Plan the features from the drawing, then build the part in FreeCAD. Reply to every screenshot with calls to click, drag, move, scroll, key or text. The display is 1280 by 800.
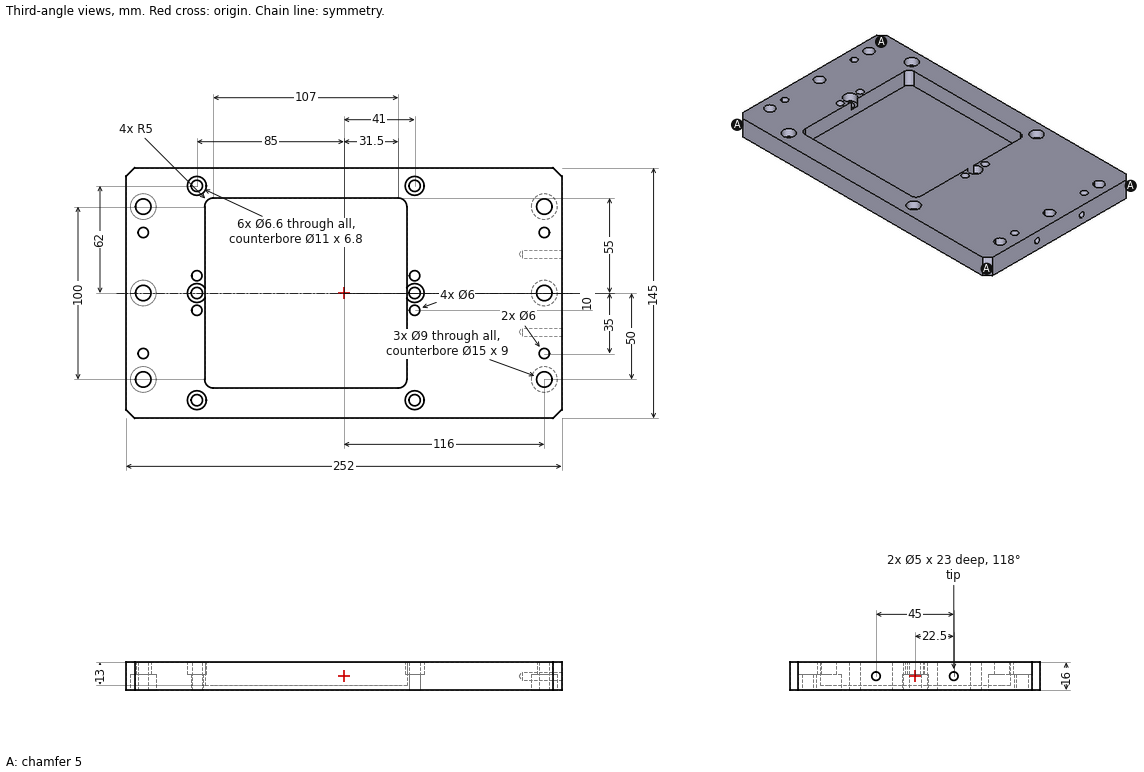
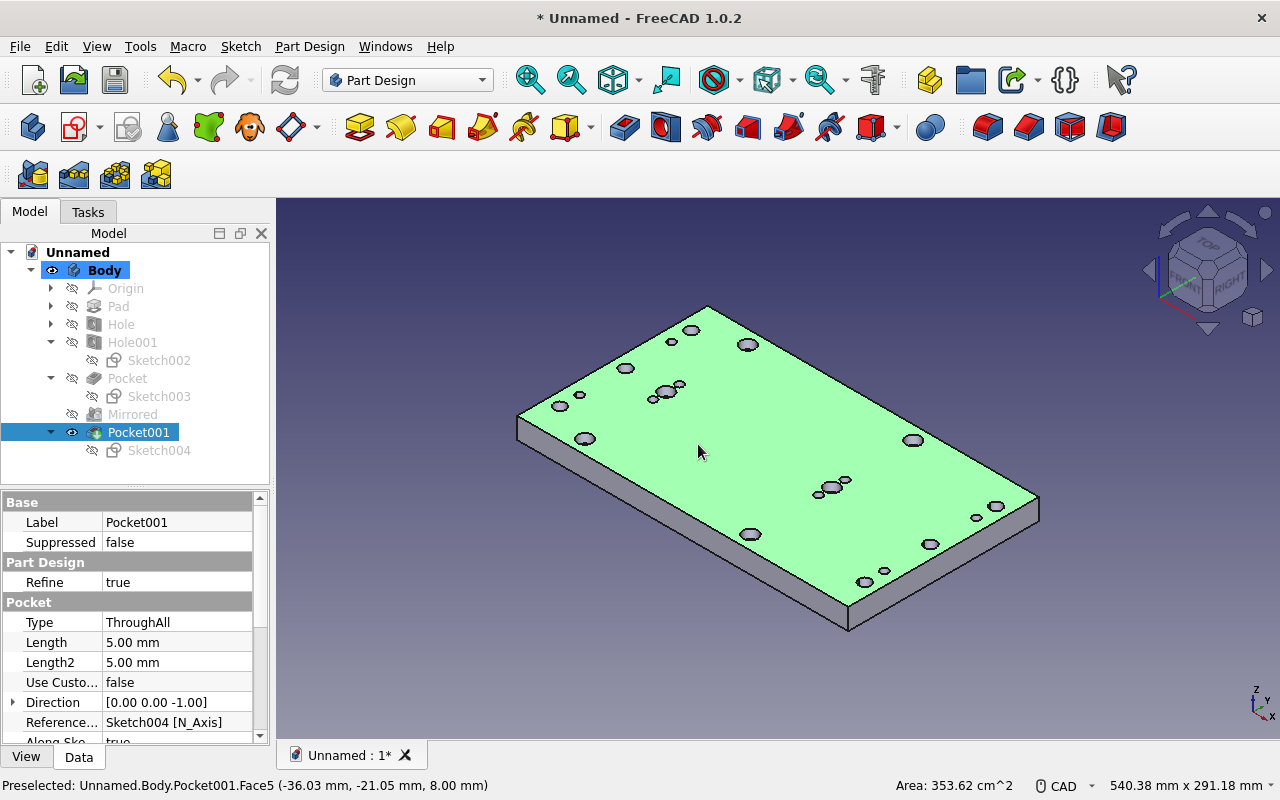
click(74, 128)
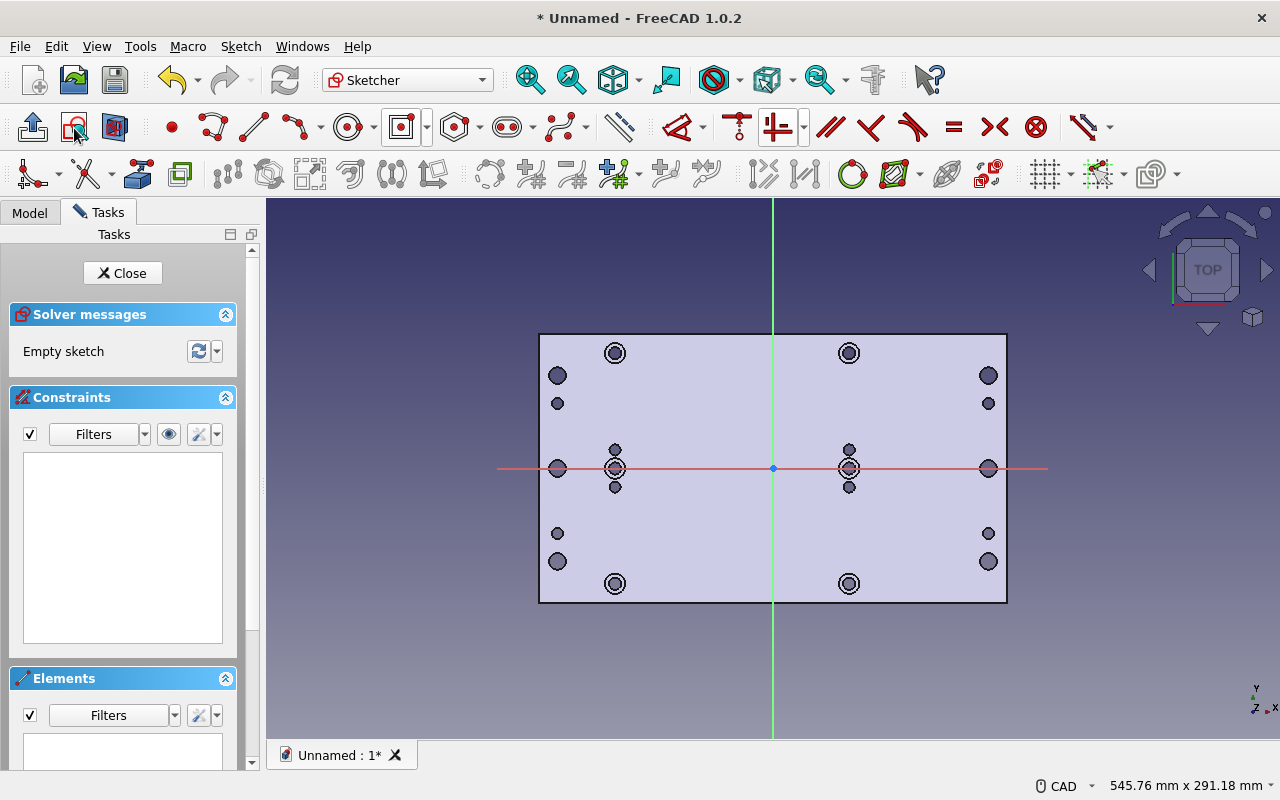
scroll(766, 468, up, 3)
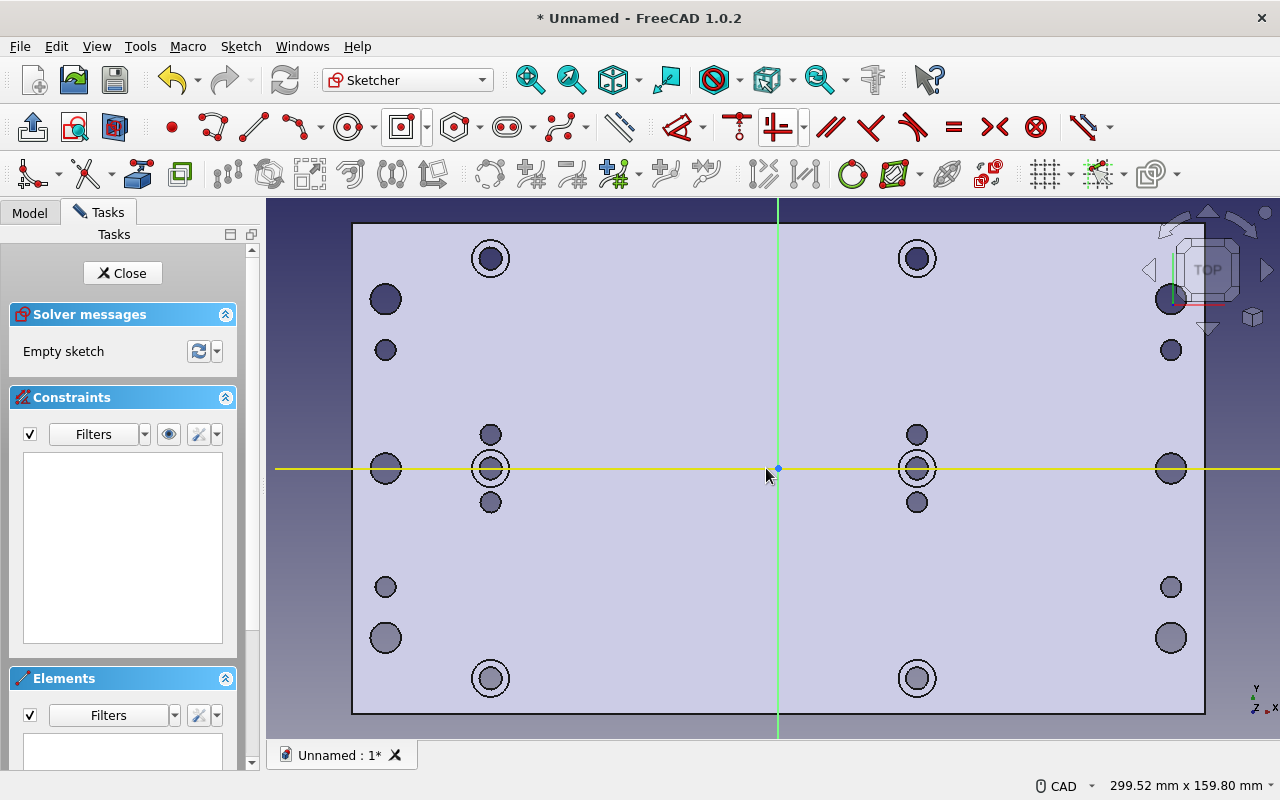
click(254, 128)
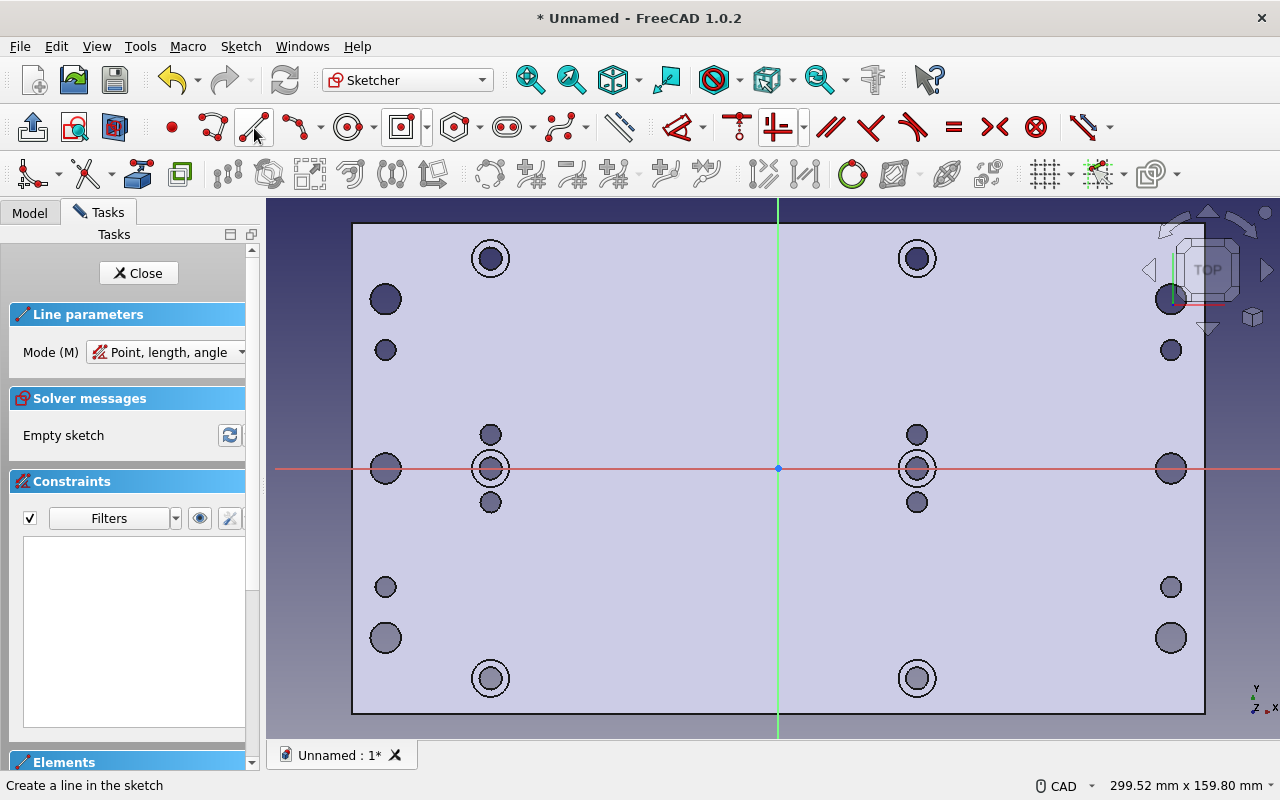
click(885, 282)
click(523, 282)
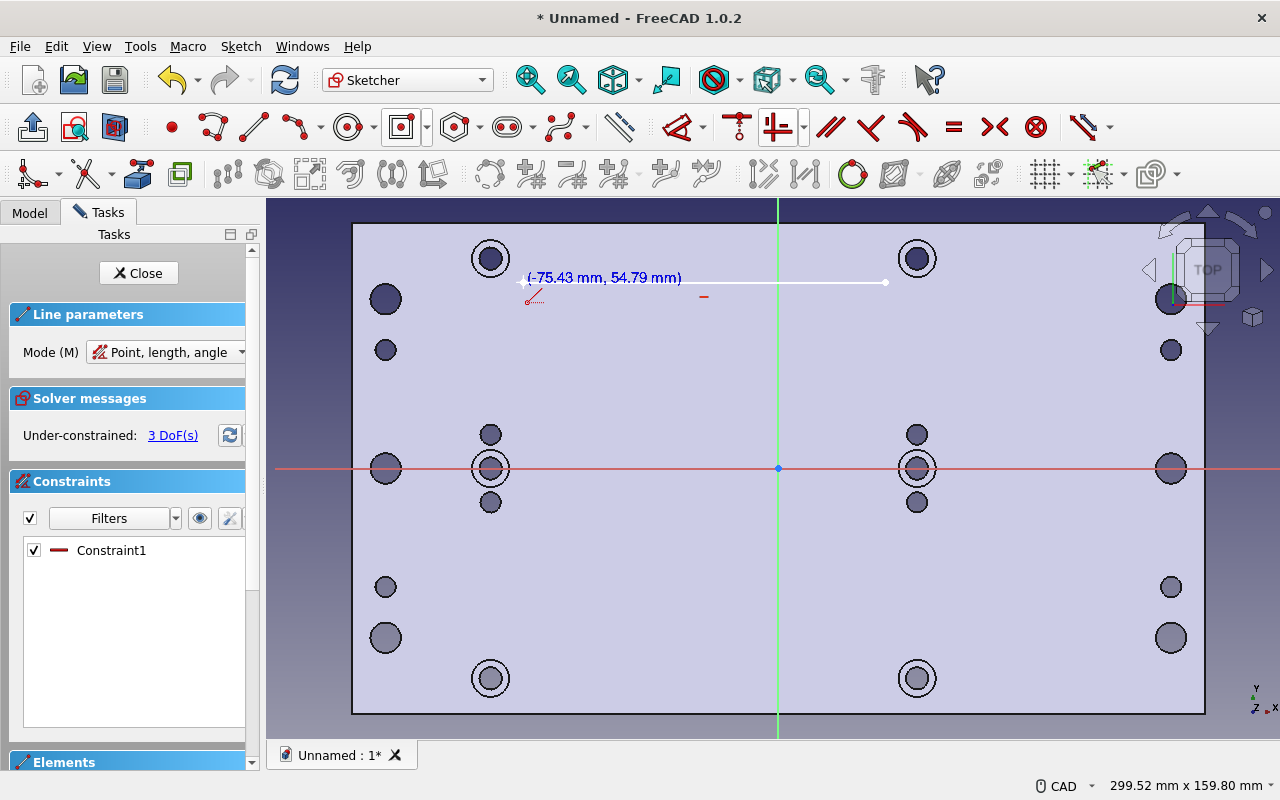
click(506, 299)
click(506, 638)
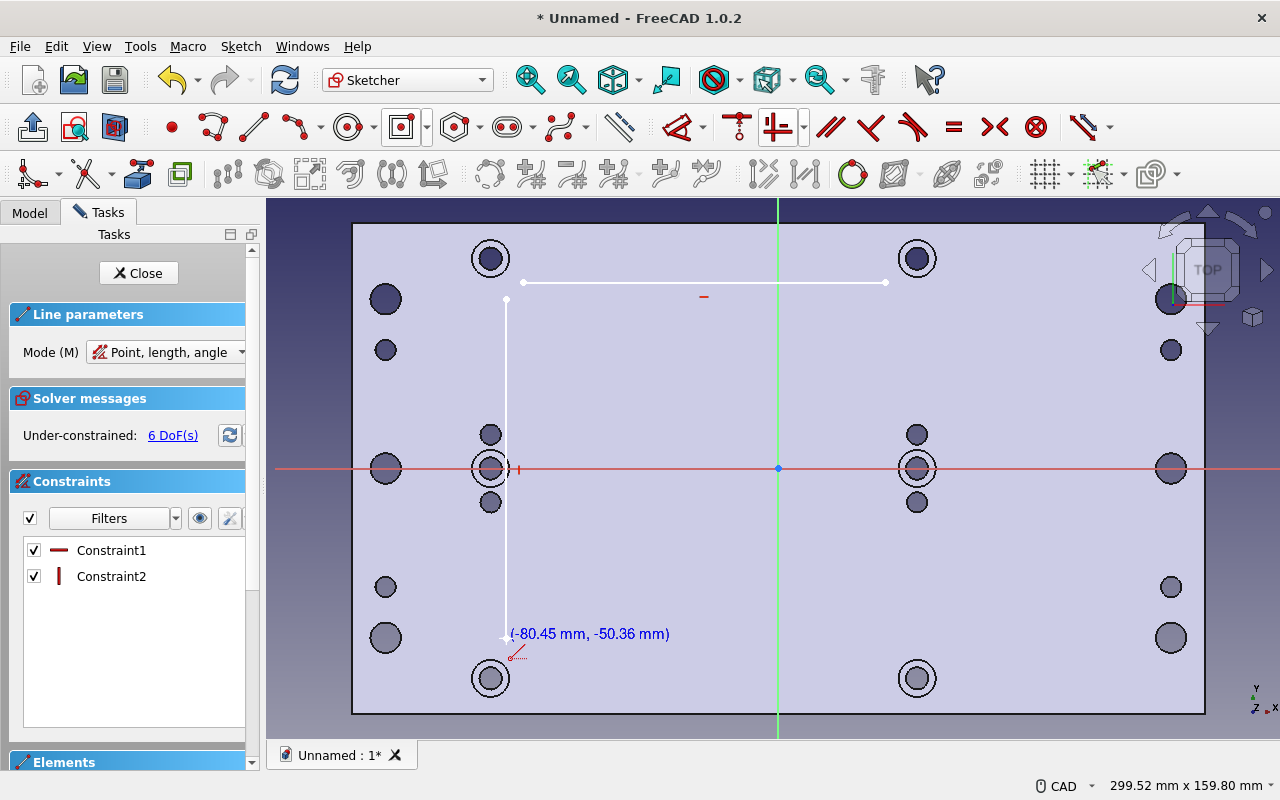
click(523, 655)
click(885, 655)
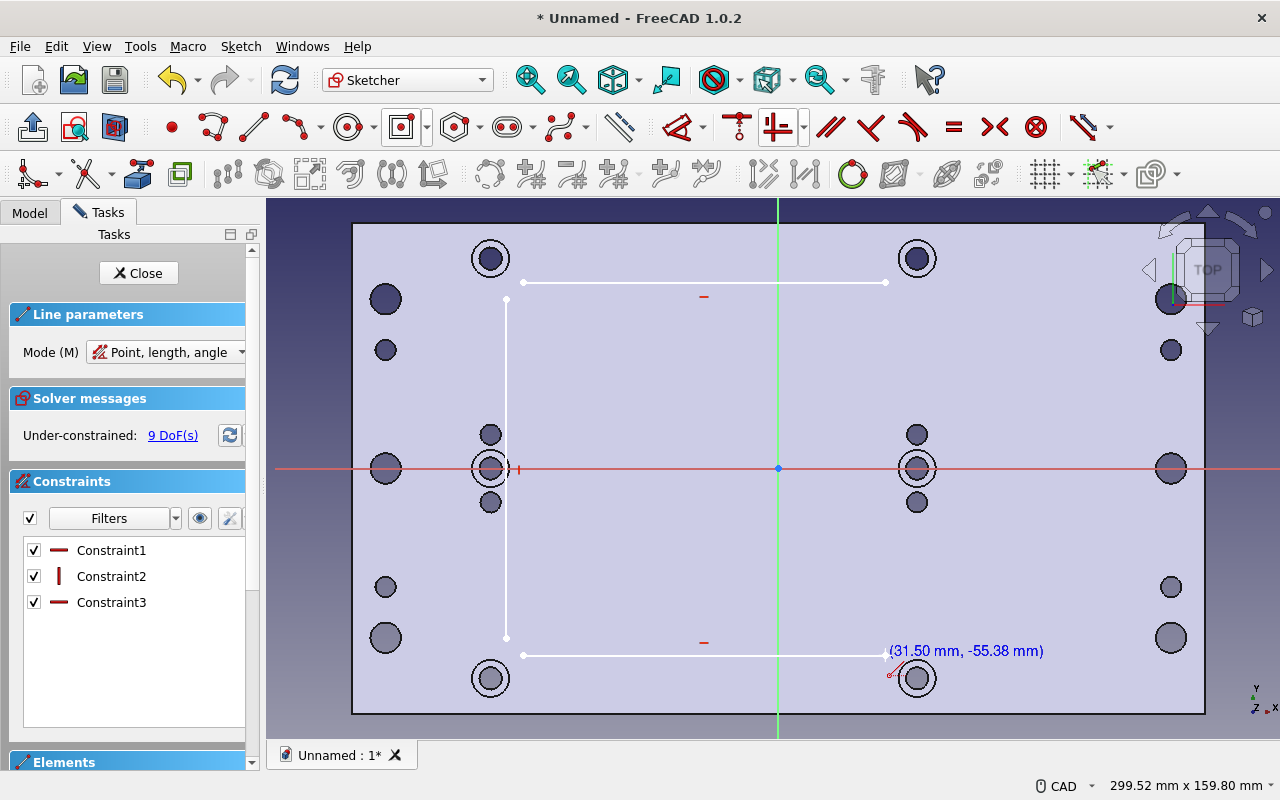
click(902, 638)
click(902, 299)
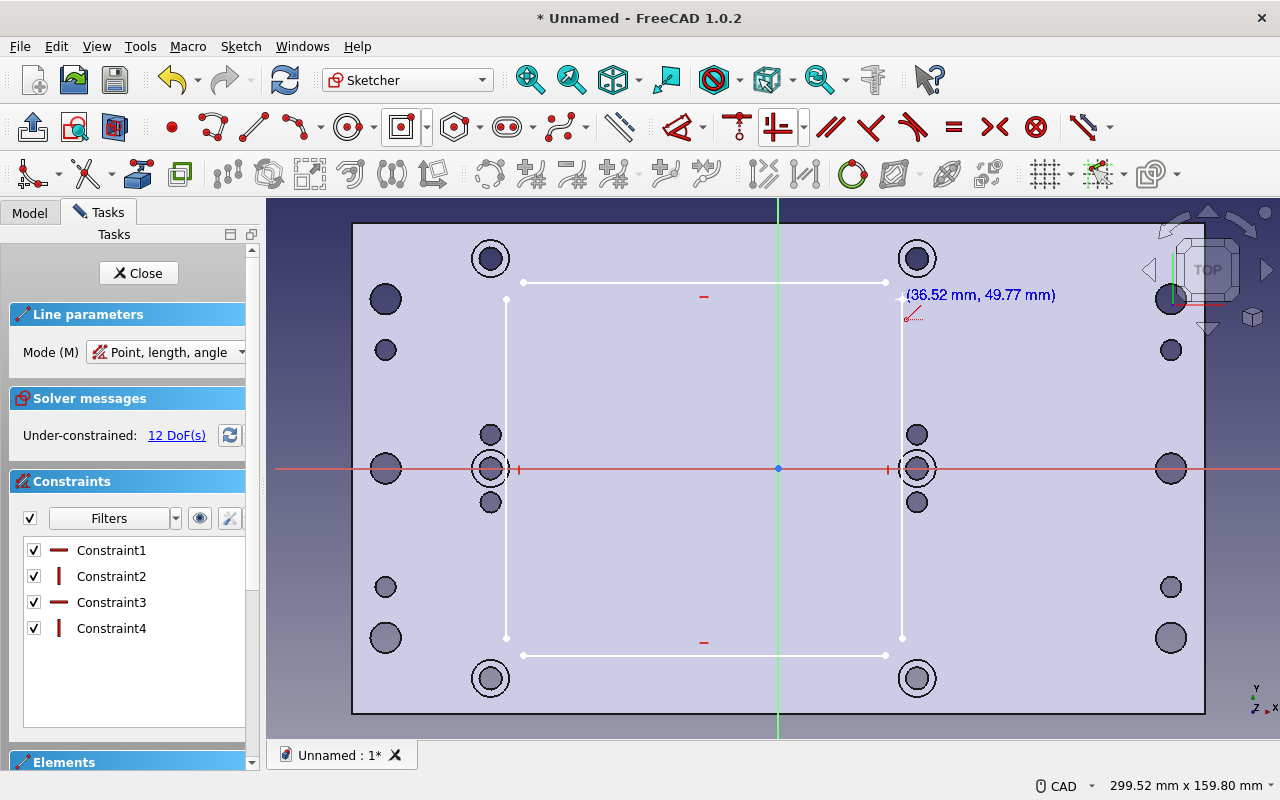
key(g)
key(3)
key(a)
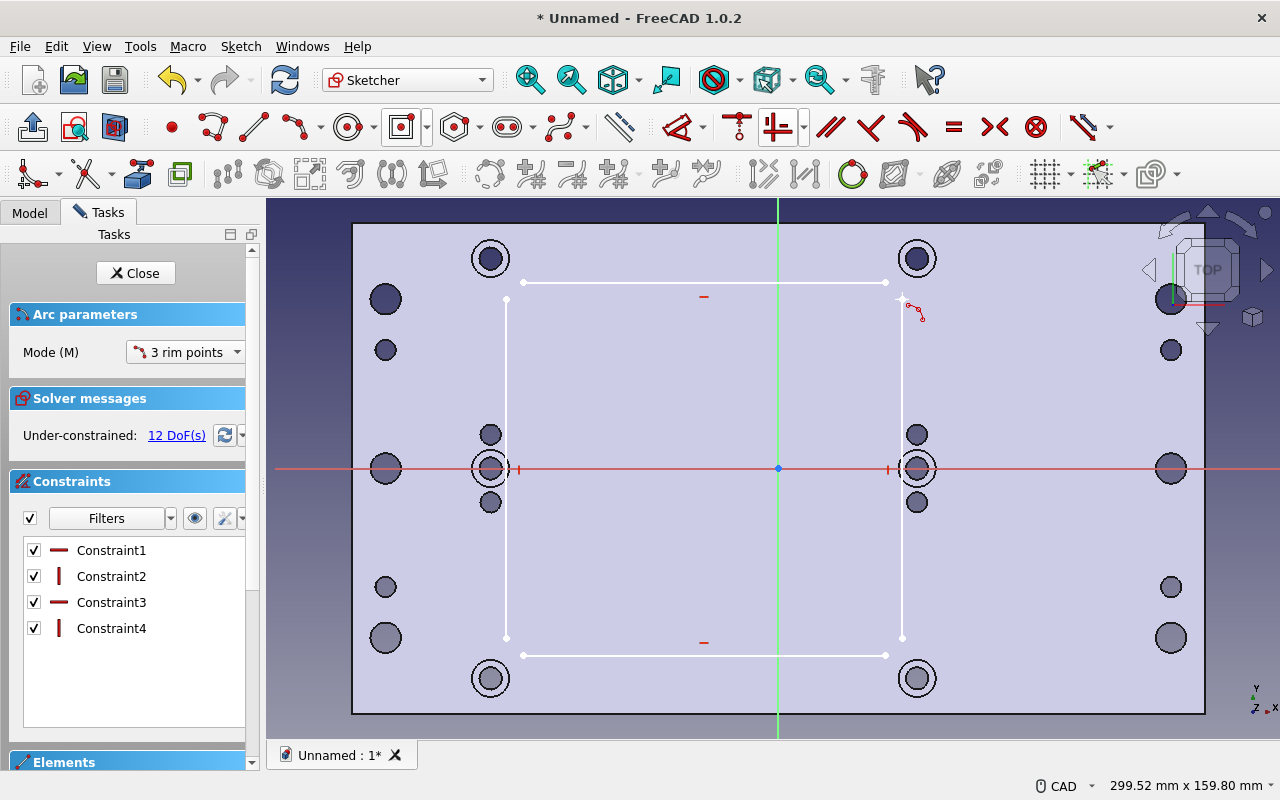
click(523, 283)
click(506, 300)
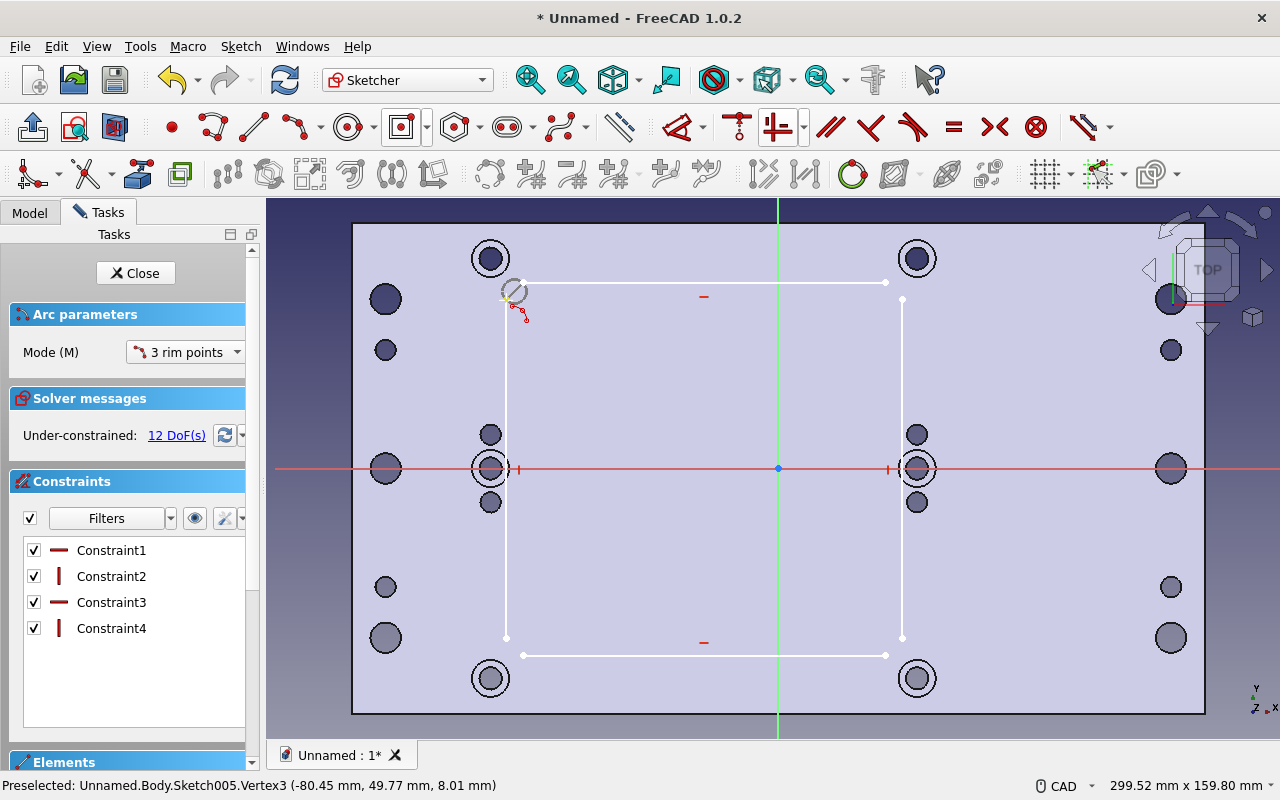
scroll(511, 287, up, 6)